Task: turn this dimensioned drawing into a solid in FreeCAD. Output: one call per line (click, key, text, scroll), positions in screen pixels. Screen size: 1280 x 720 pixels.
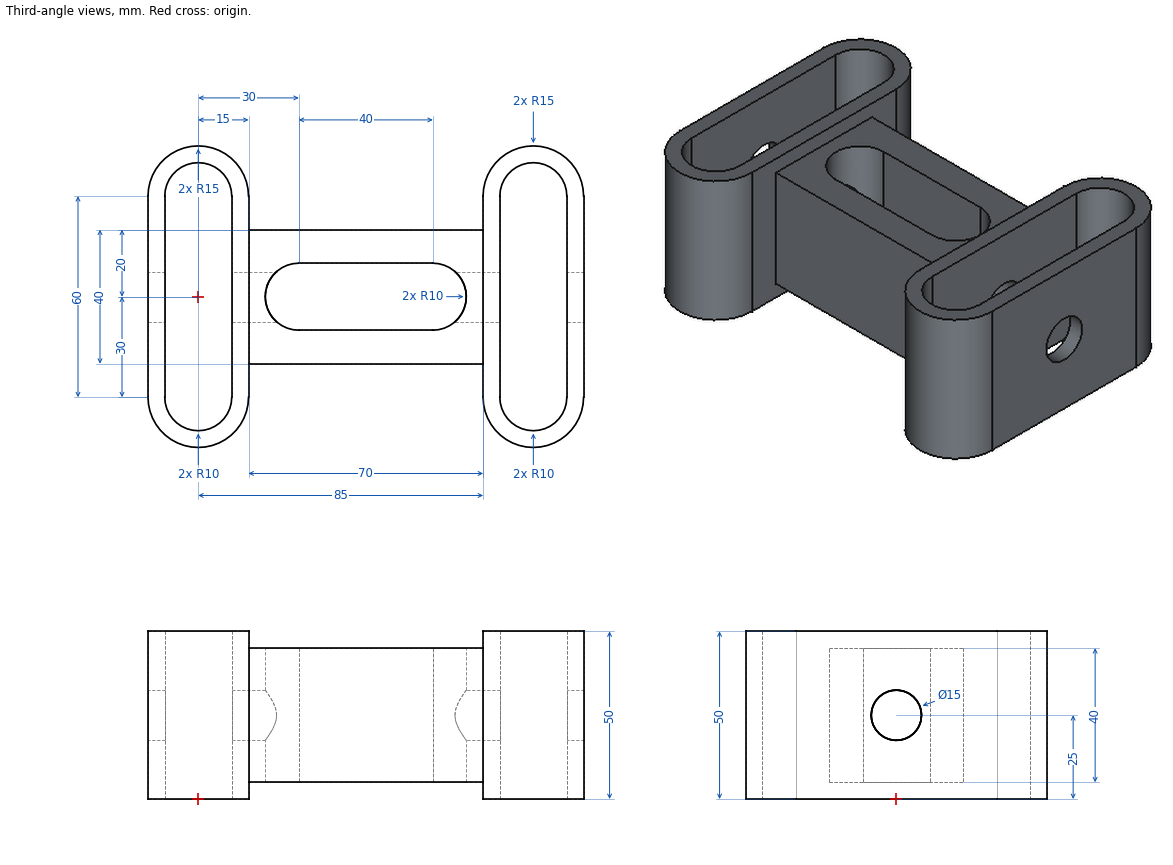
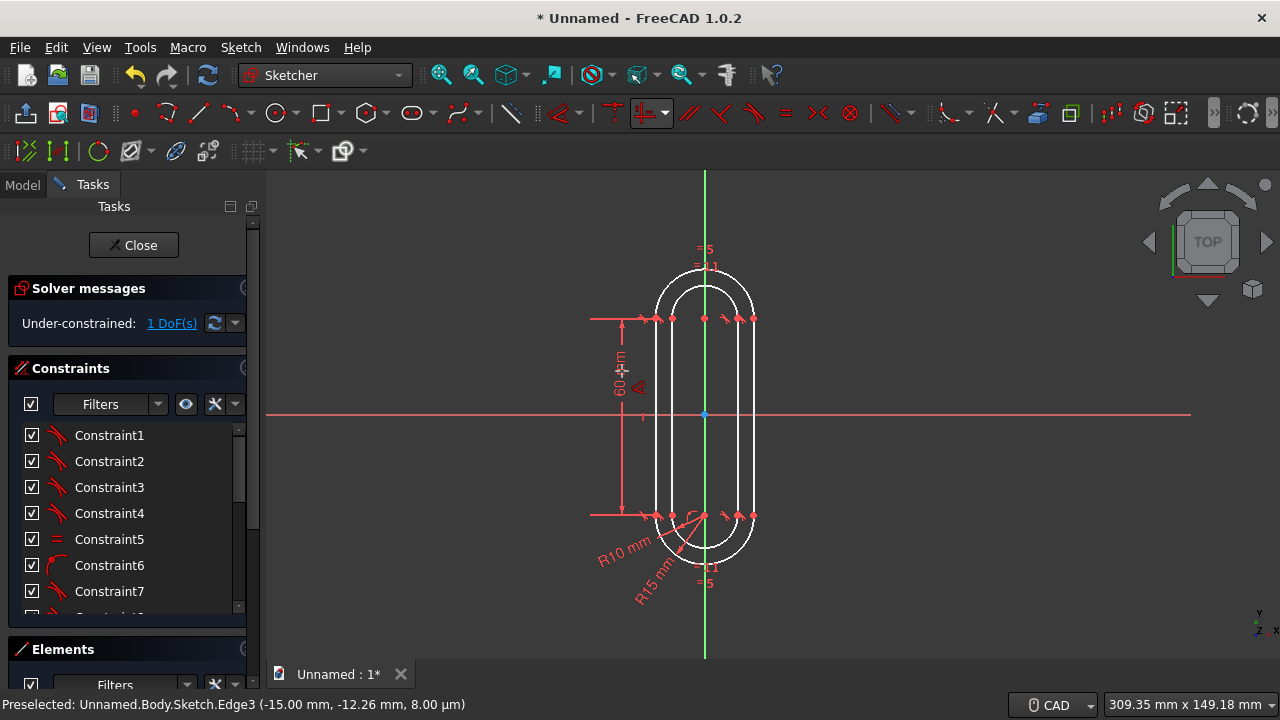
click(656, 515)
click(622, 465)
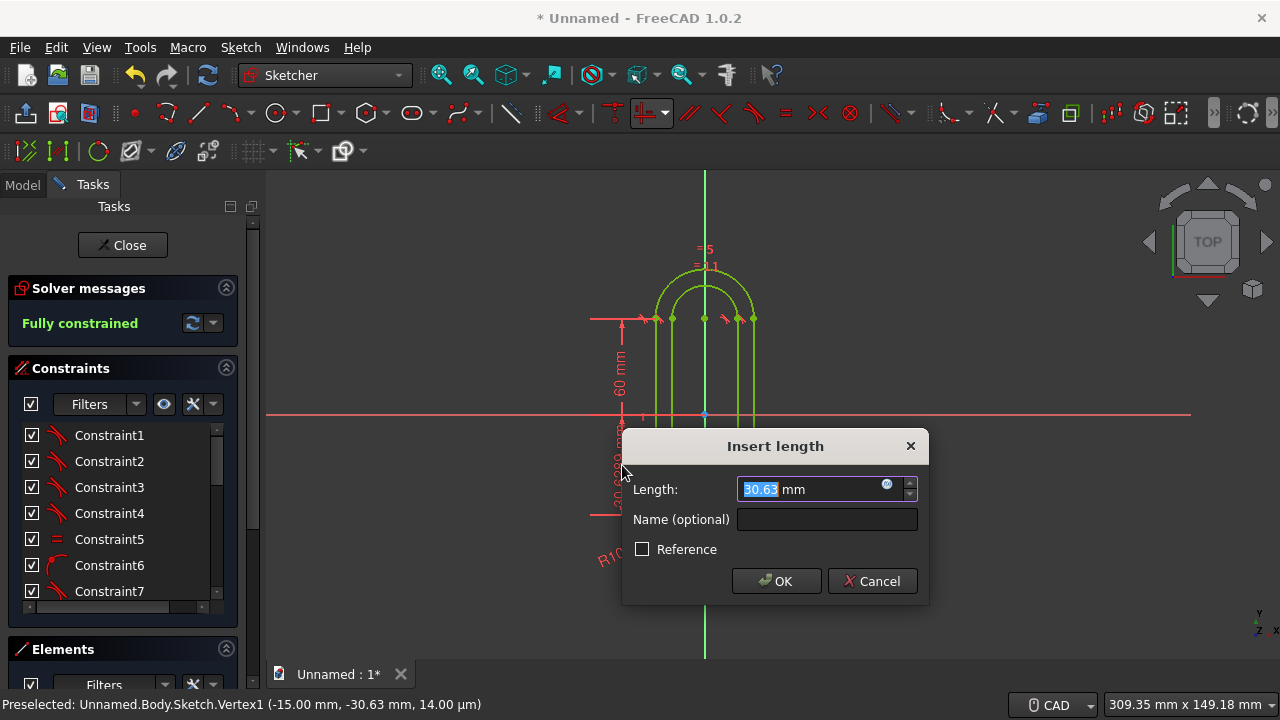
text(30)
key(Return)
key(Escape)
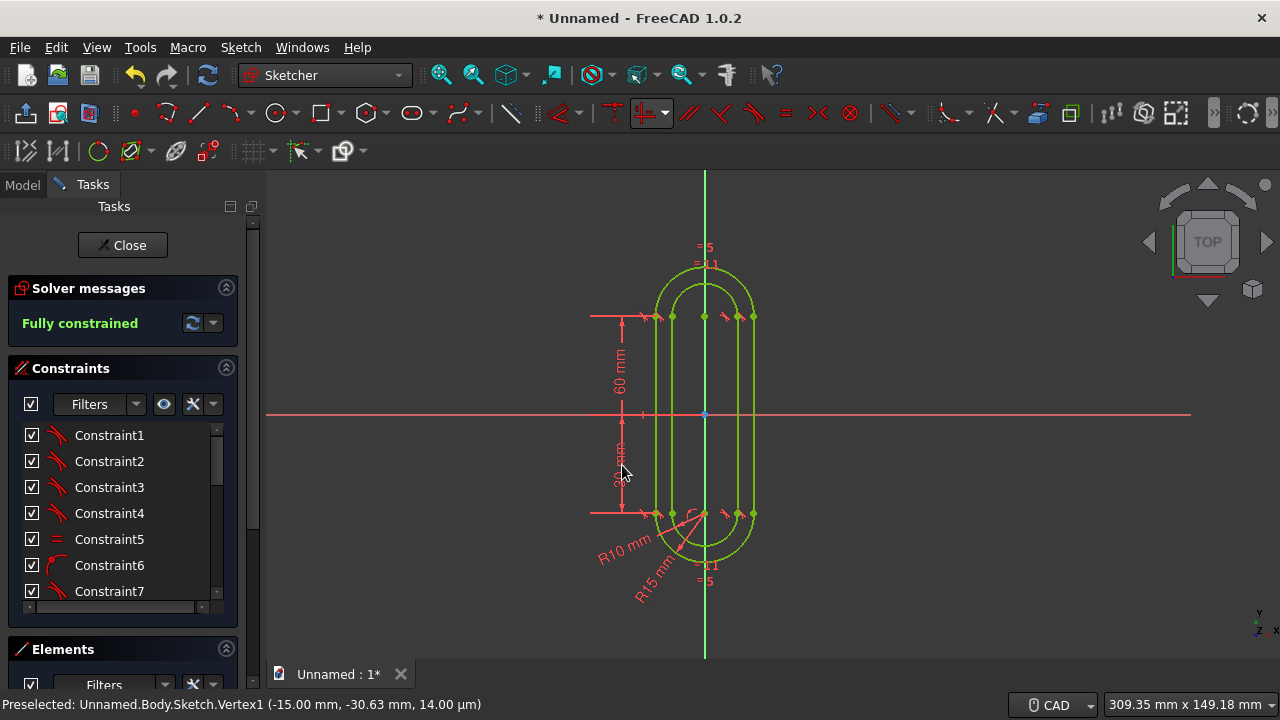
click(123, 245)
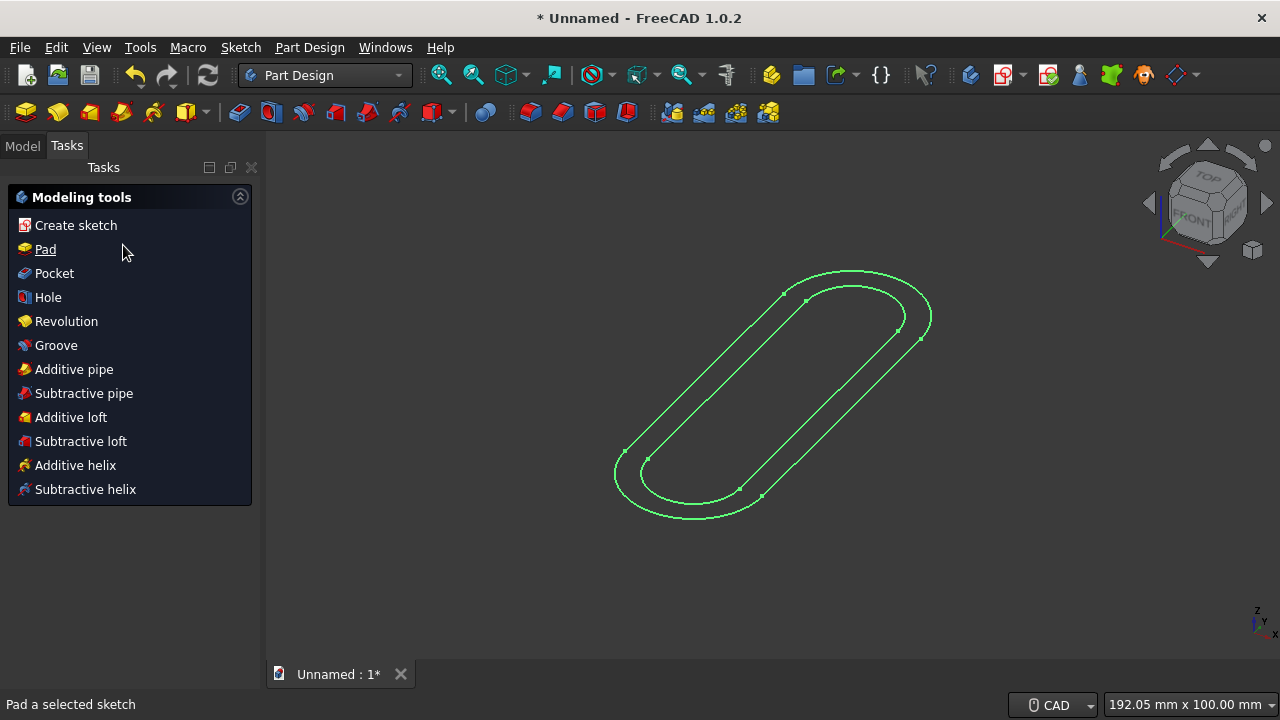
click(26, 112)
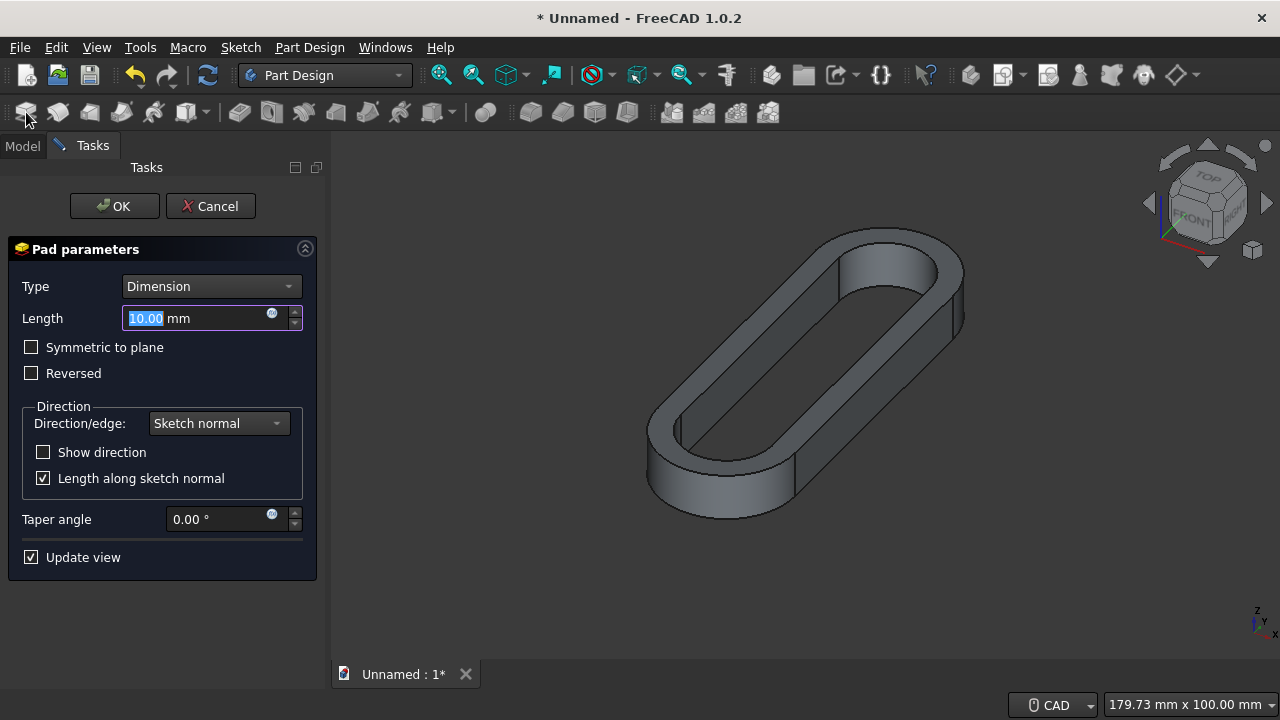
text(50)
key(Tab)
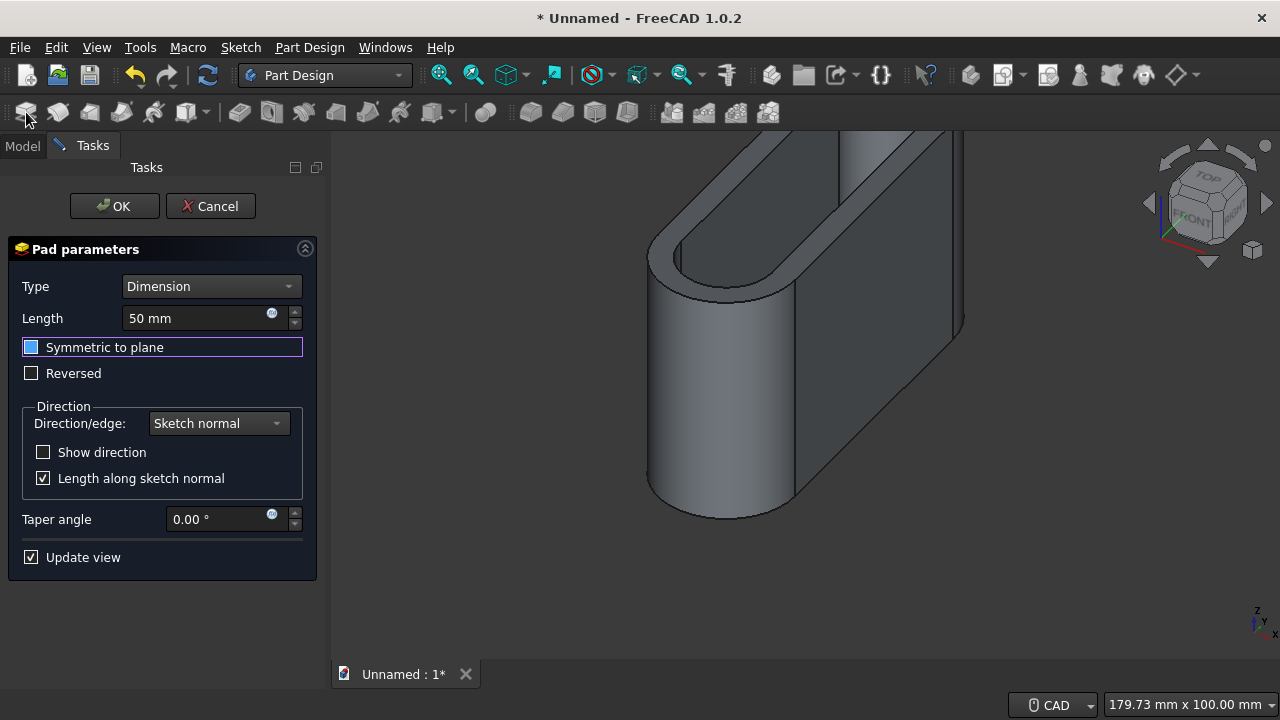
click(115, 206)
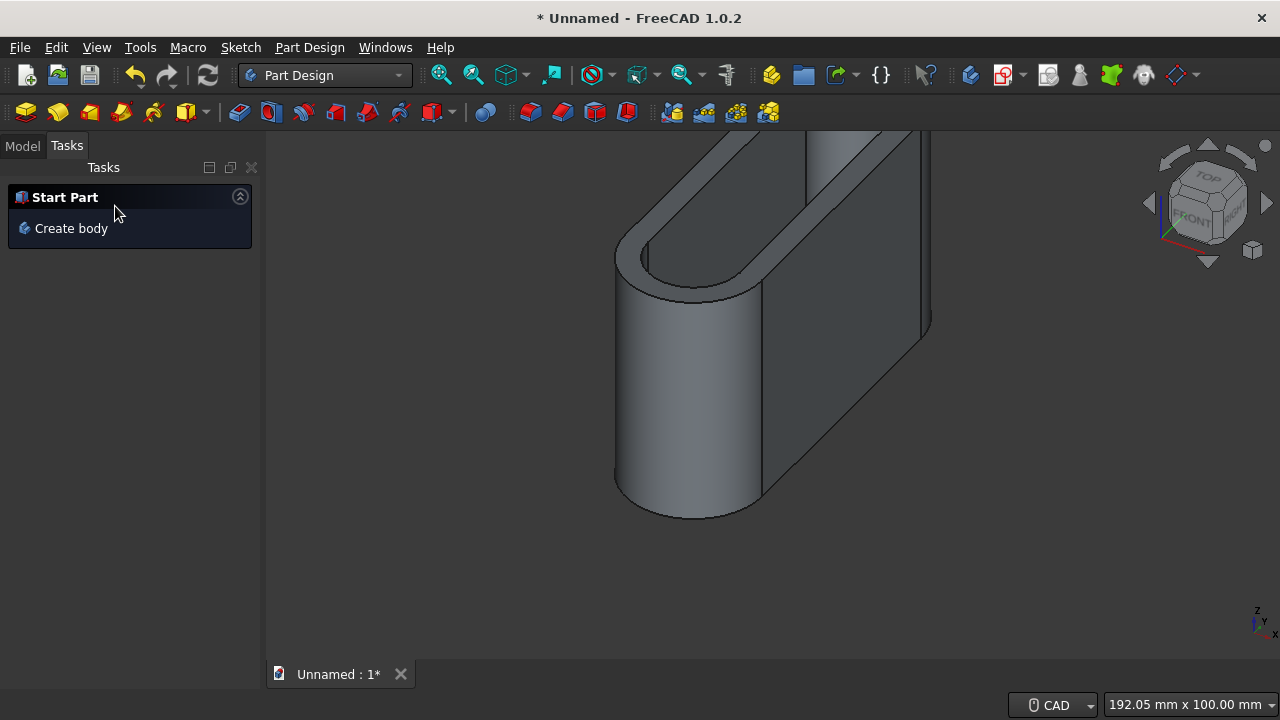
click(442, 76)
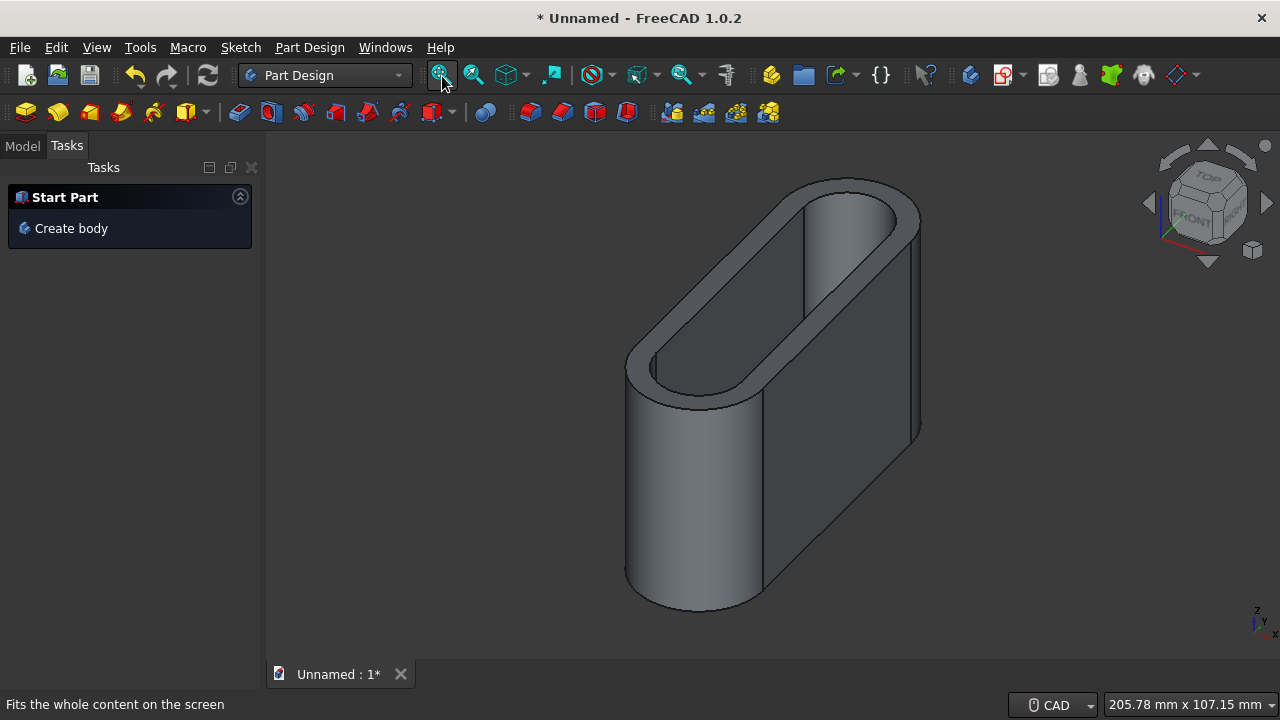
click(972, 76)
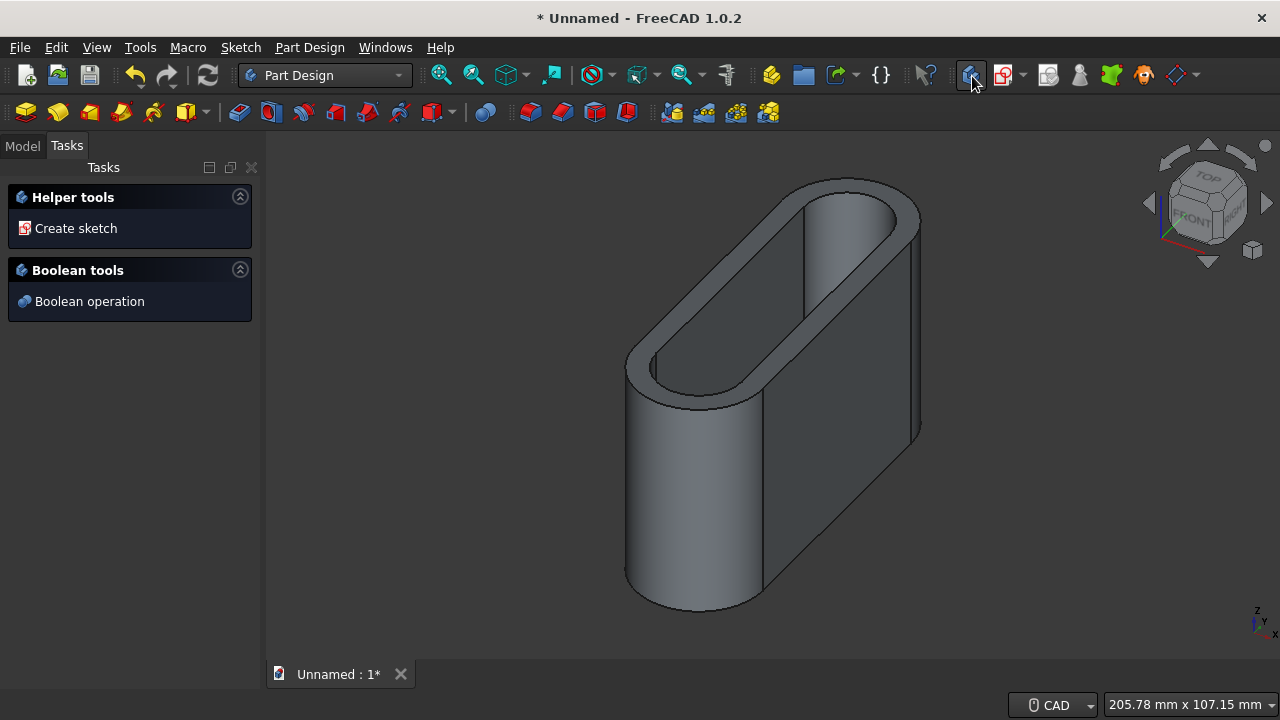
click(306, 619)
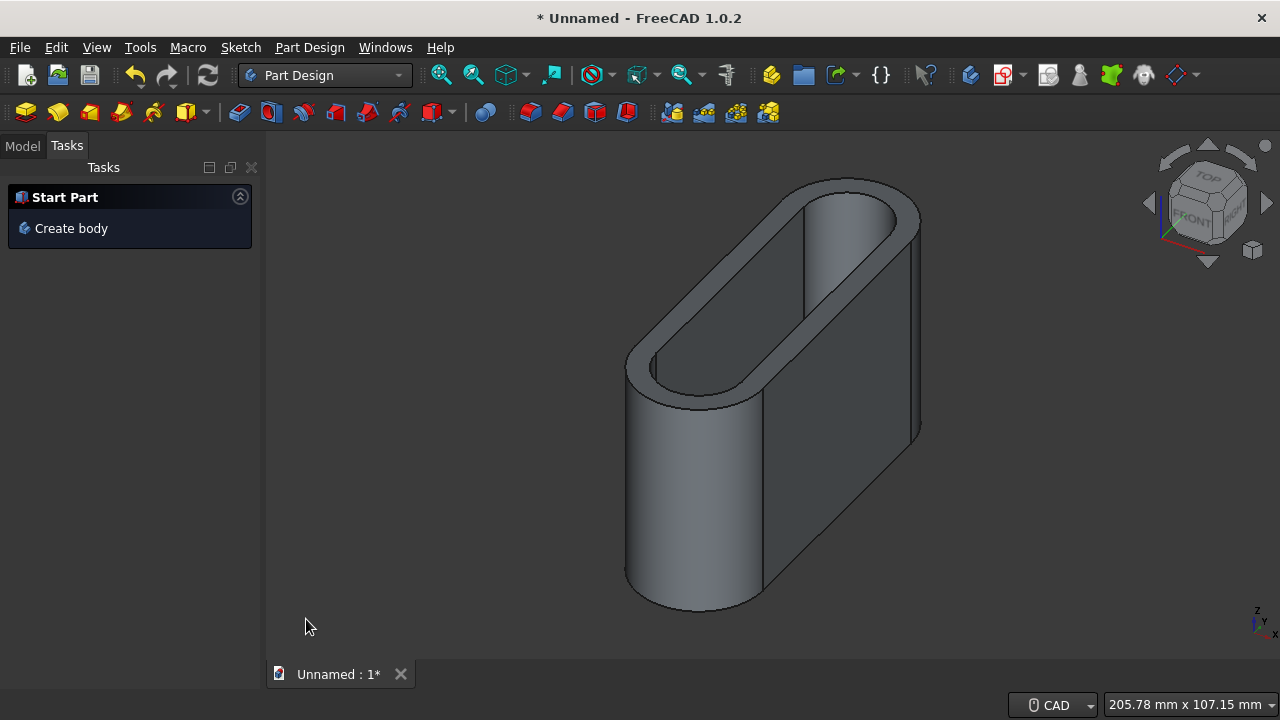
click(1004, 76)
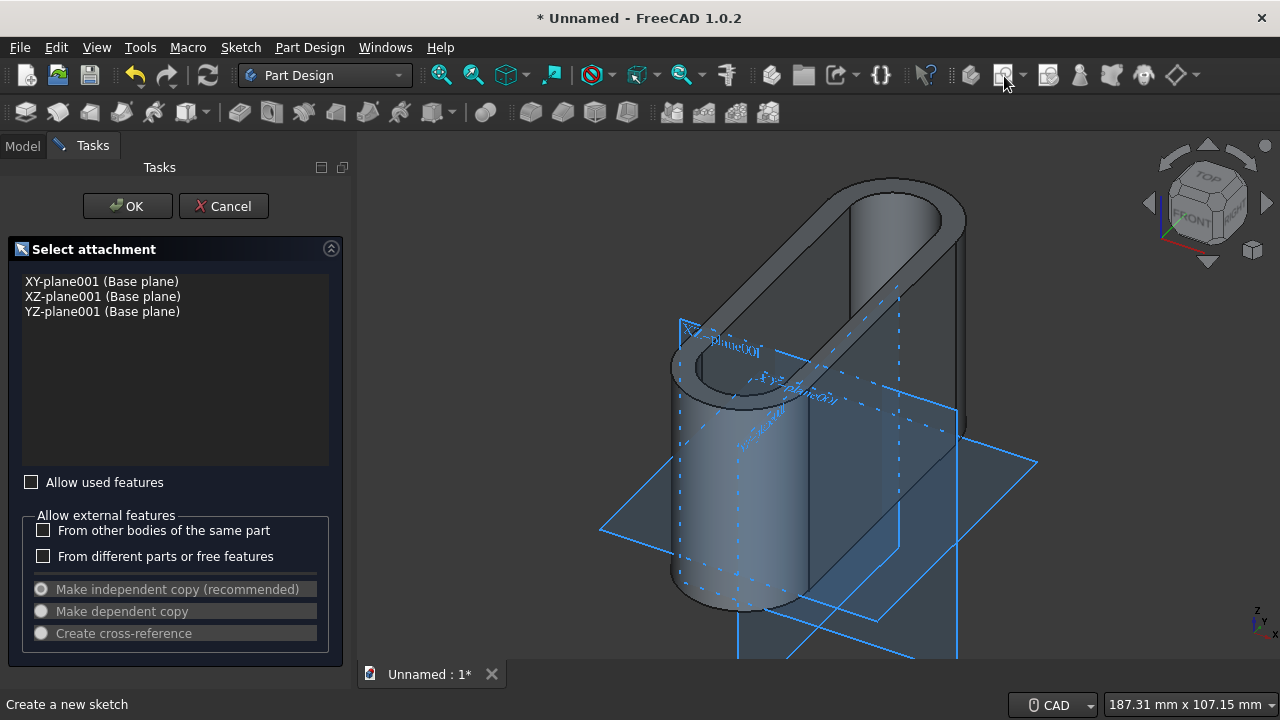
click(82, 282)